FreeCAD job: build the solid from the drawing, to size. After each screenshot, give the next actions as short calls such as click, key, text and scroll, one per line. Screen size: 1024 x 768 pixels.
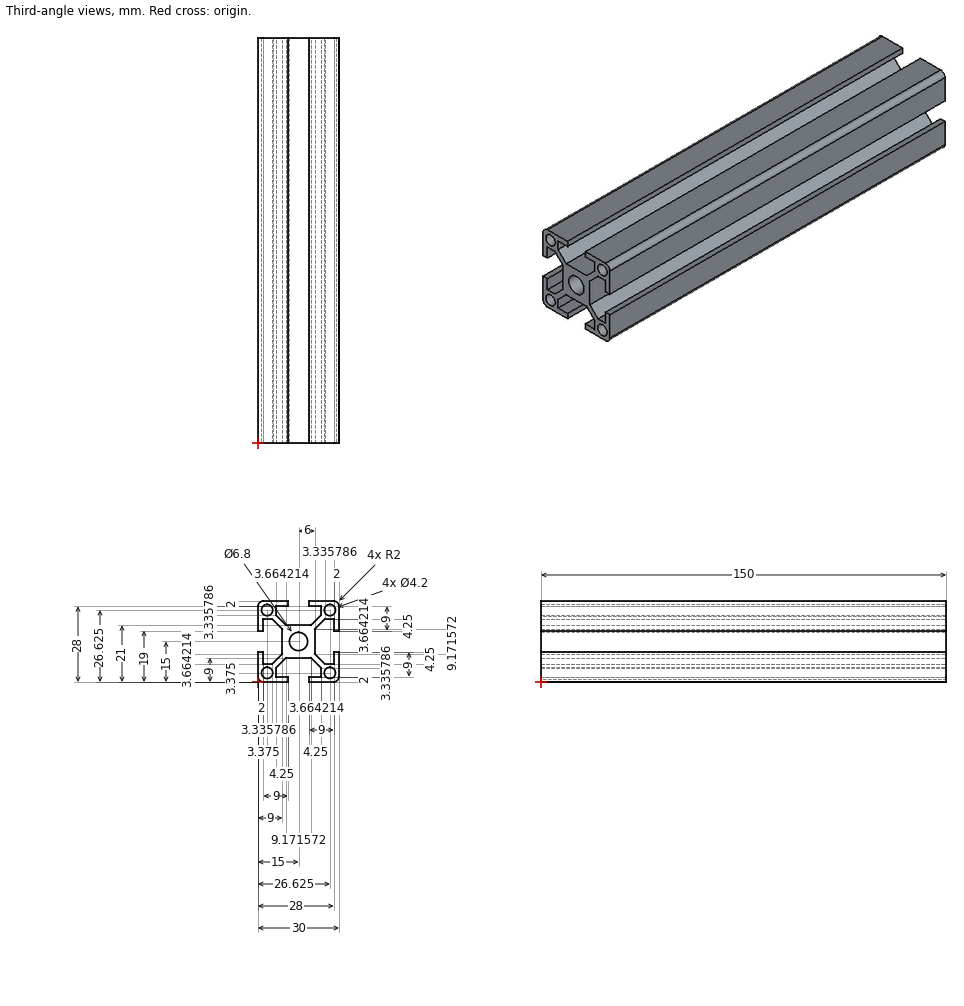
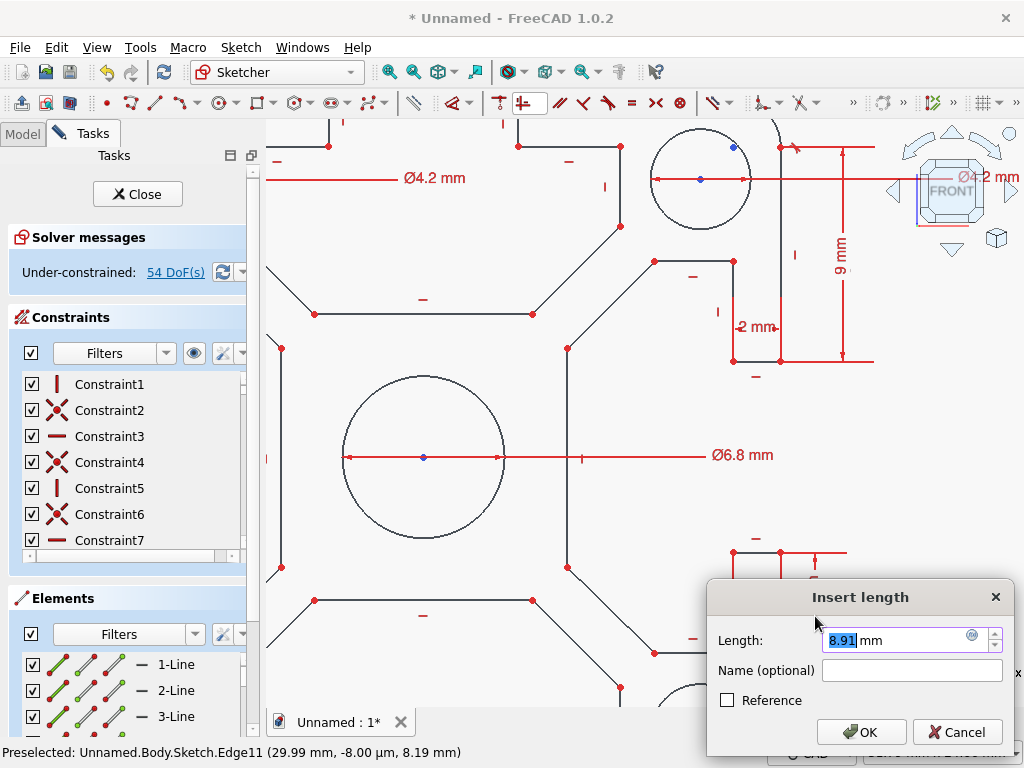
text(9)
key(Return)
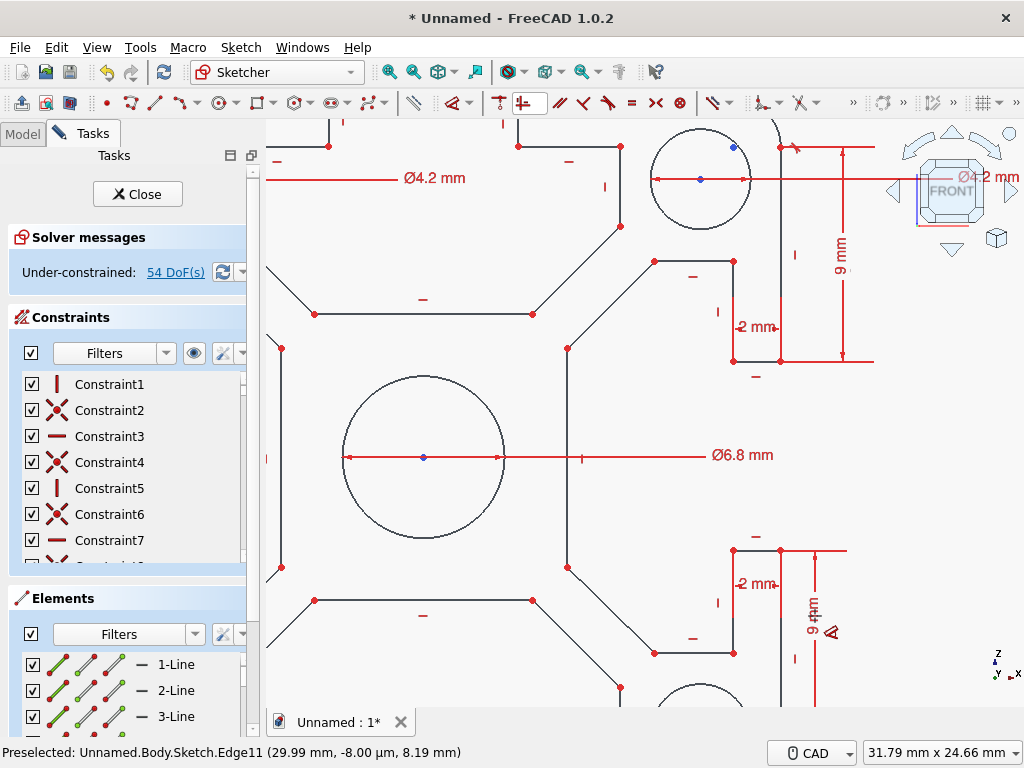
scroll(763, 361, down, 3)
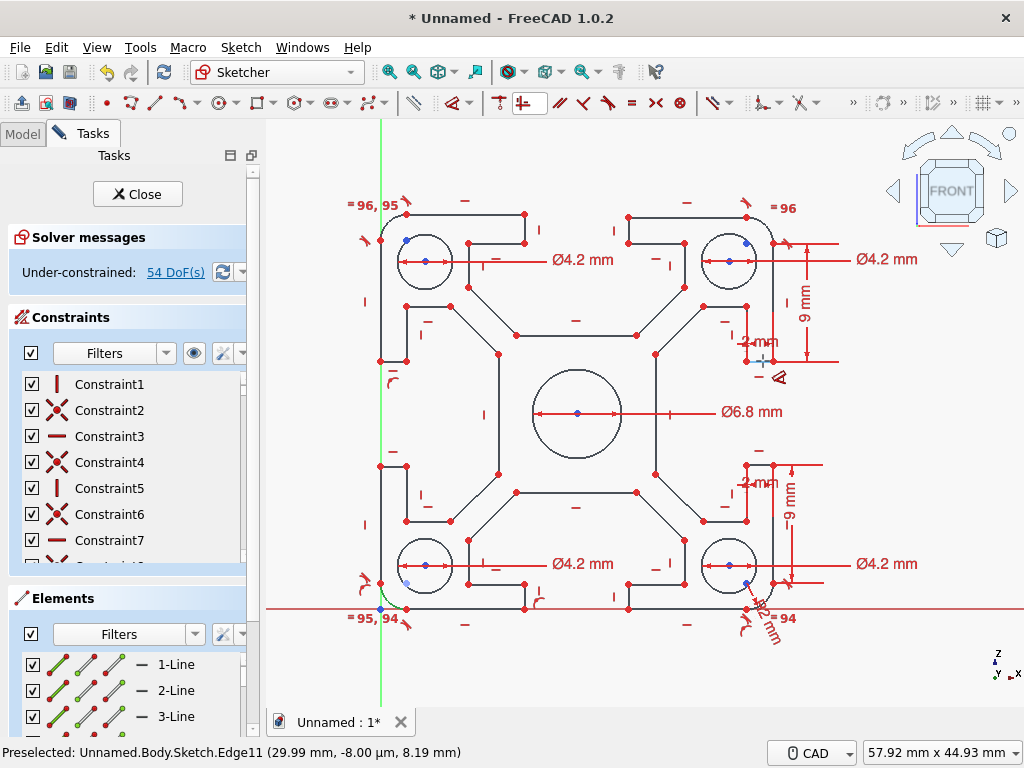
click(711, 609)
click(688, 643)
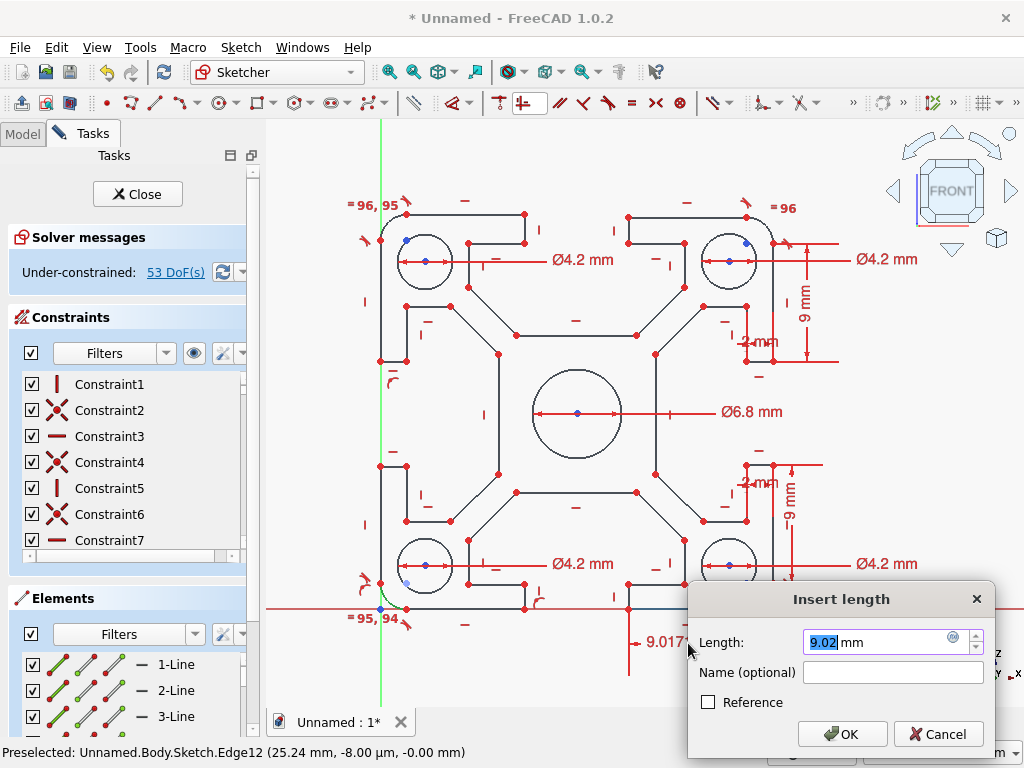
text(9)
key(Return)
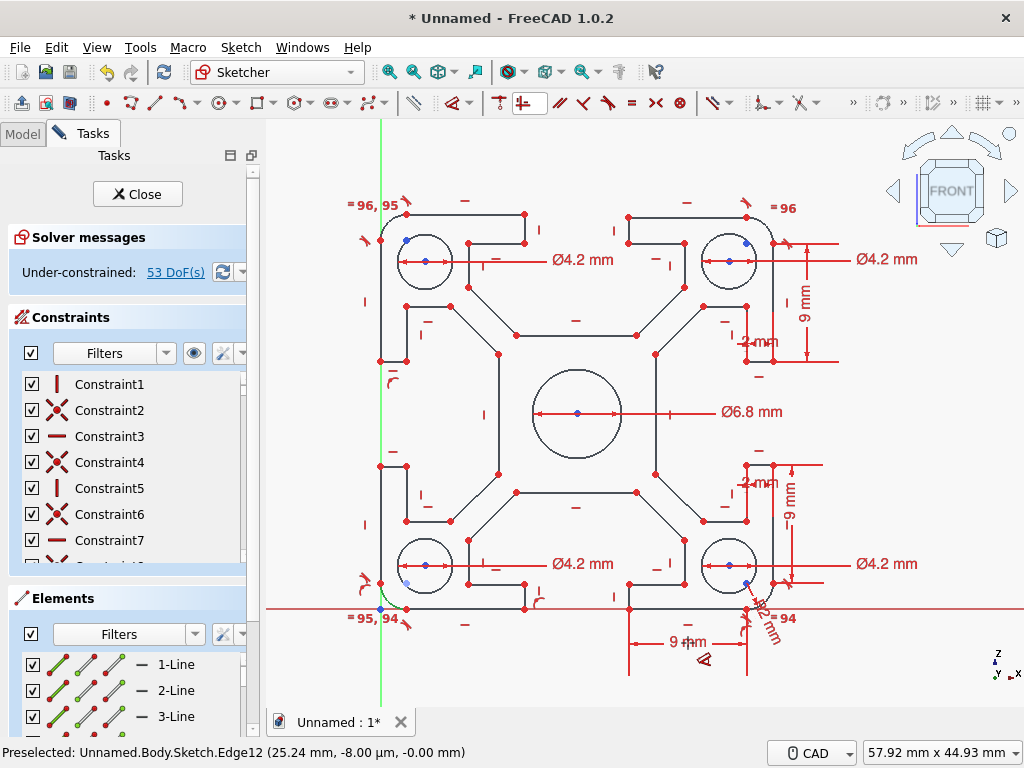
scroll(629, 599, up, 3)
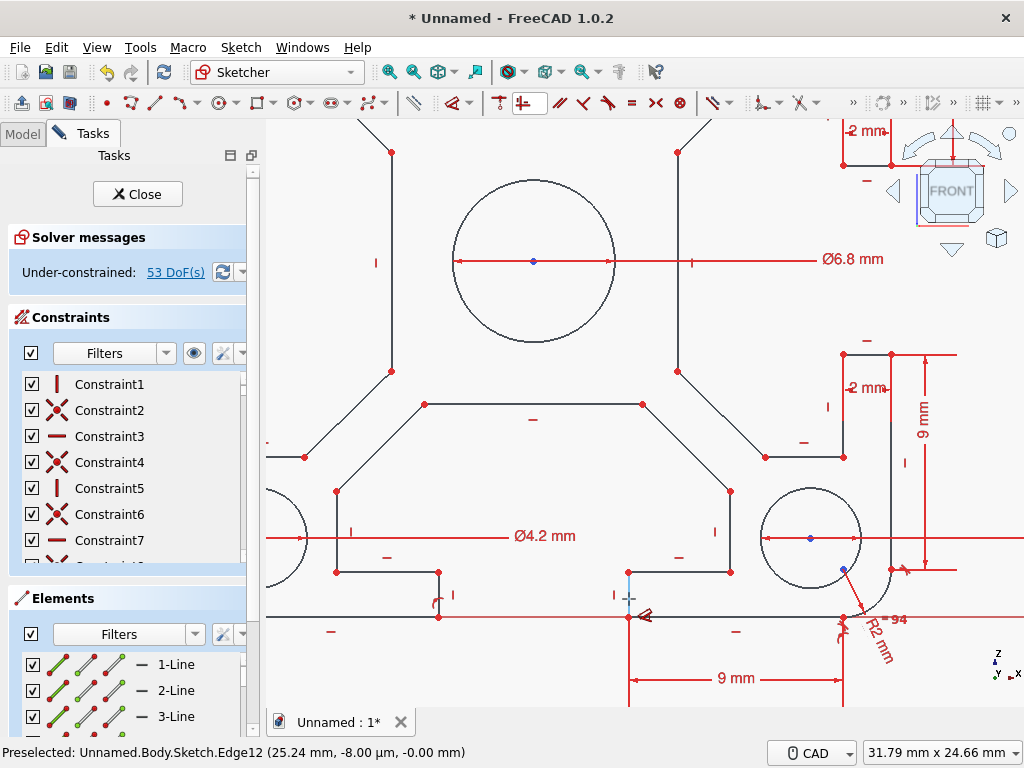
click(629, 599)
click(663, 595)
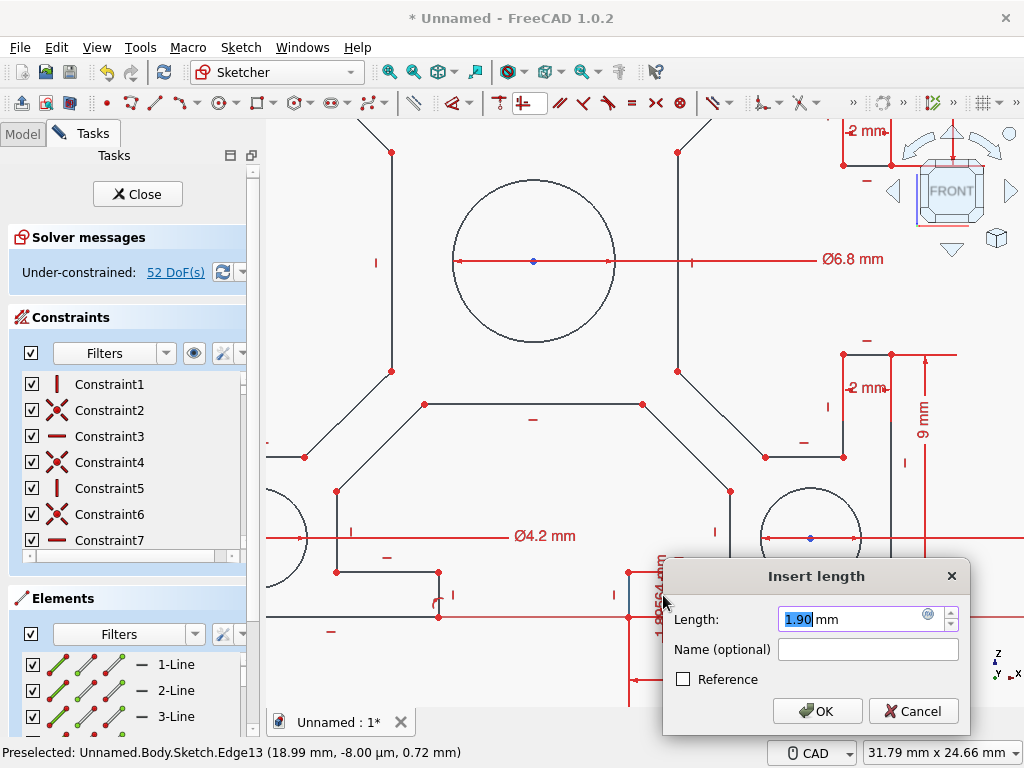
text(2)
key(Return)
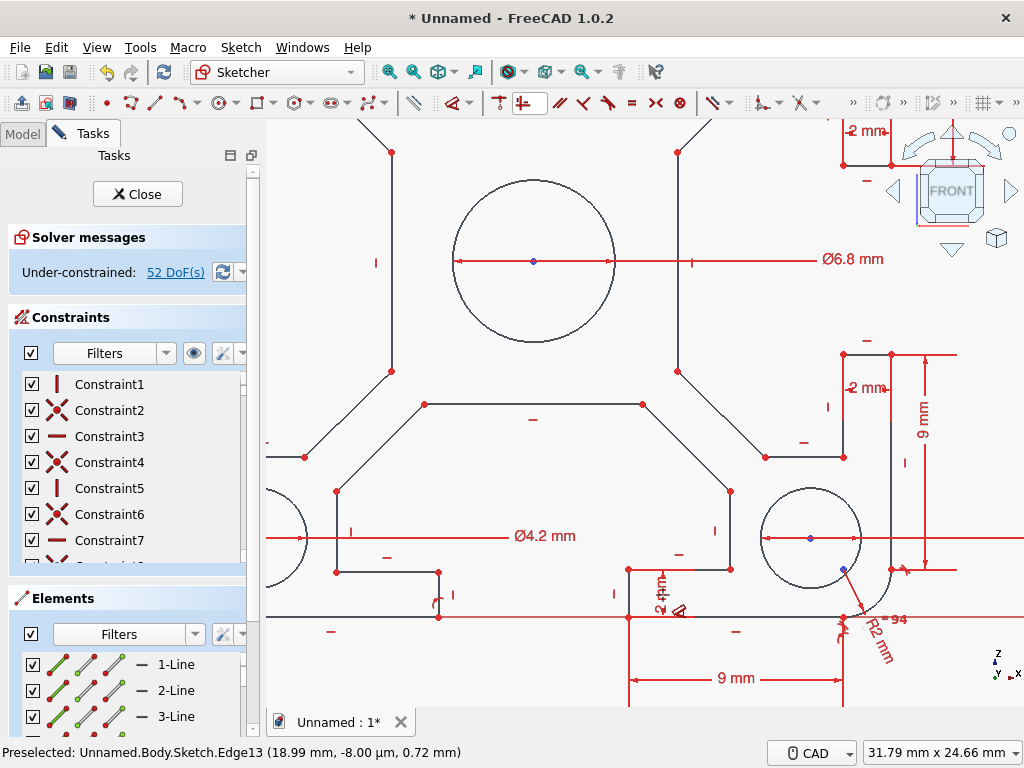
click(439, 586)
click(405, 595)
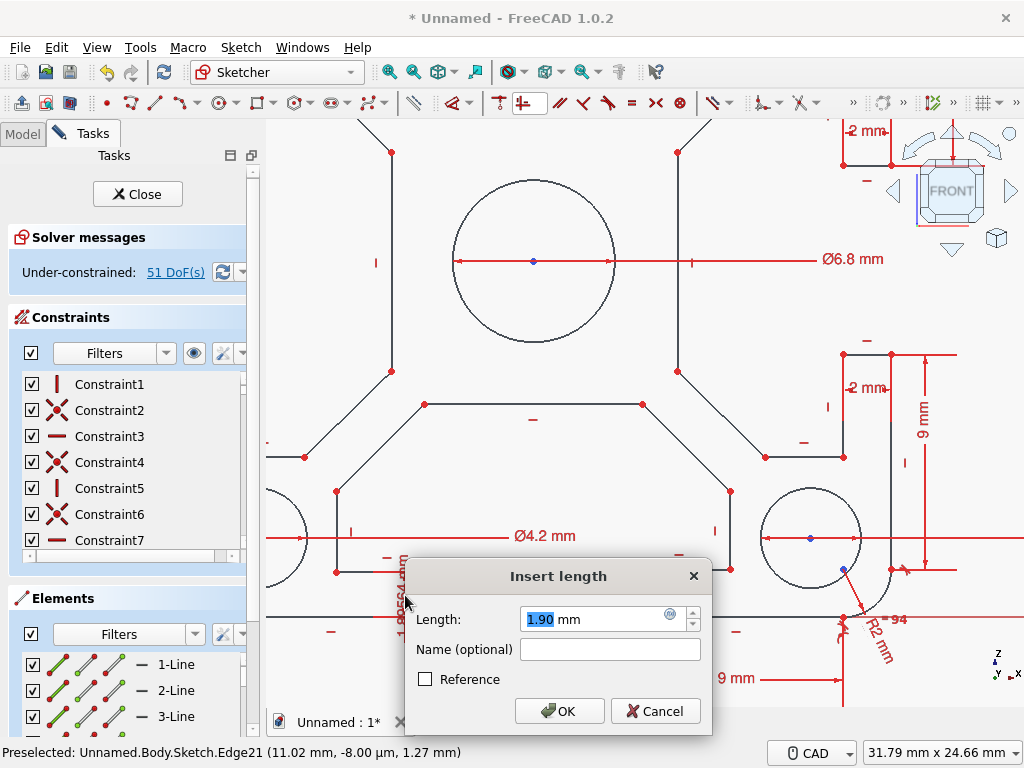
text(2)
key(Return)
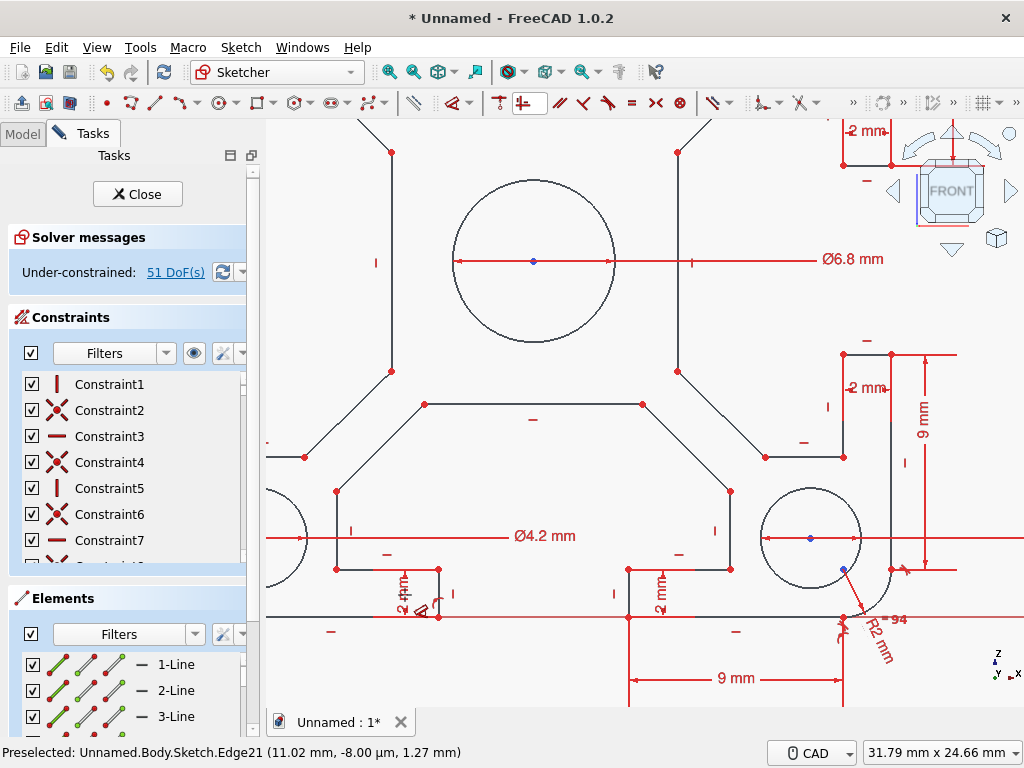
click(374, 617)
click(366, 651)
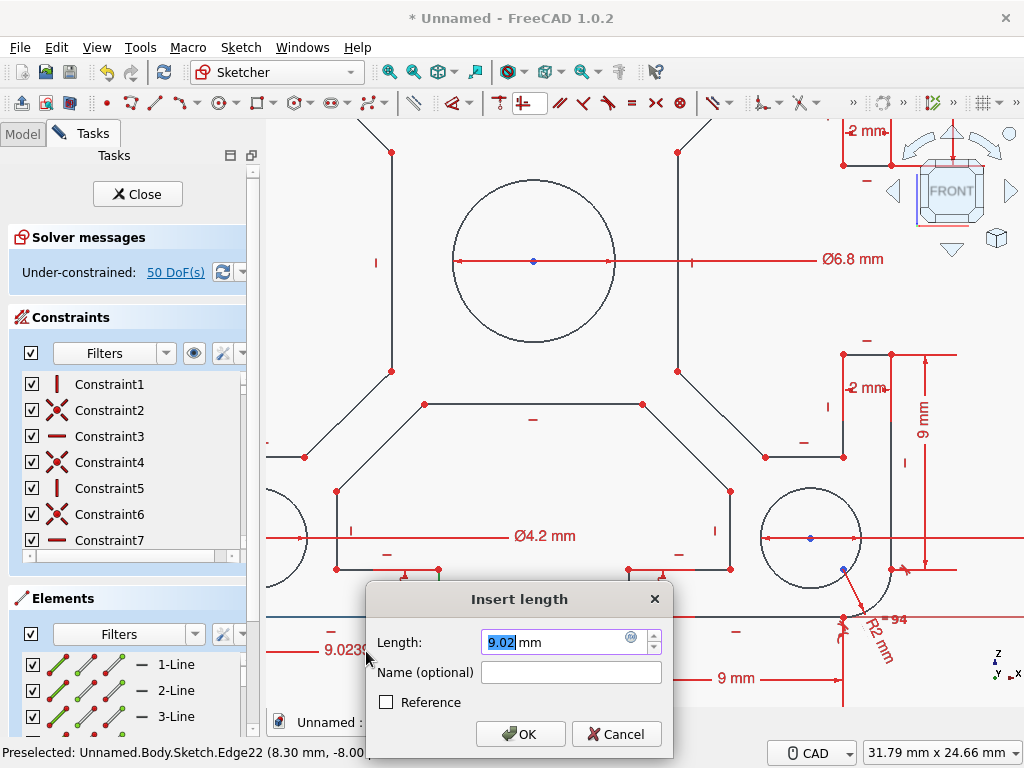
text(9)
key(Return)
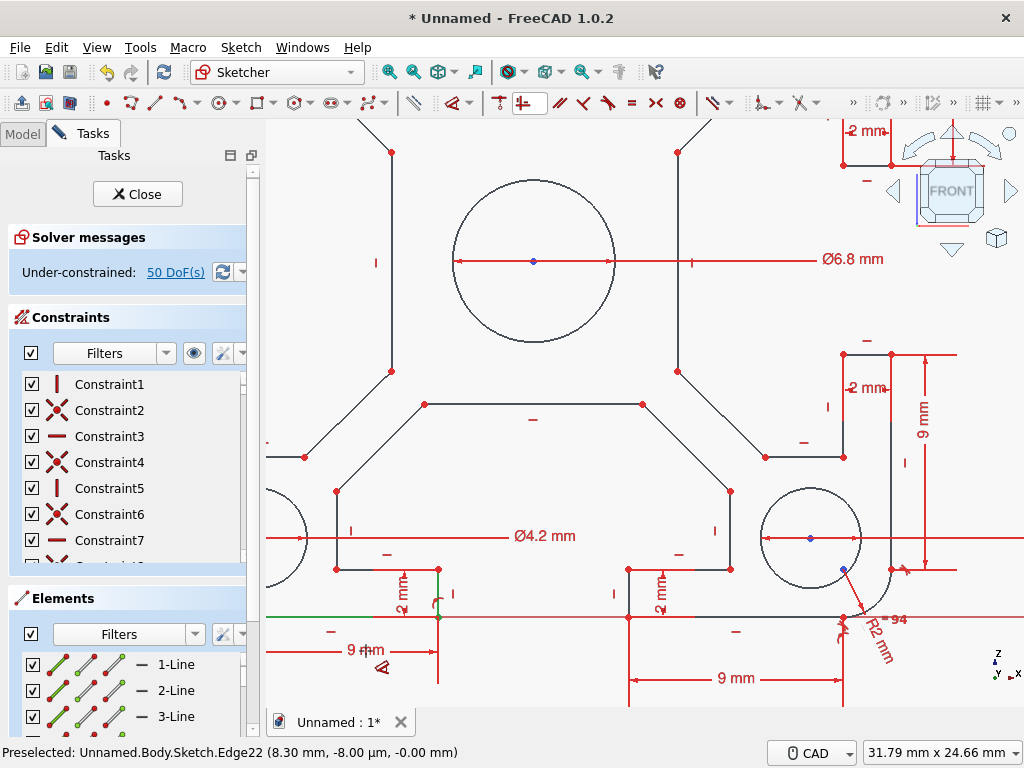
scroll(628, 600, down, 3)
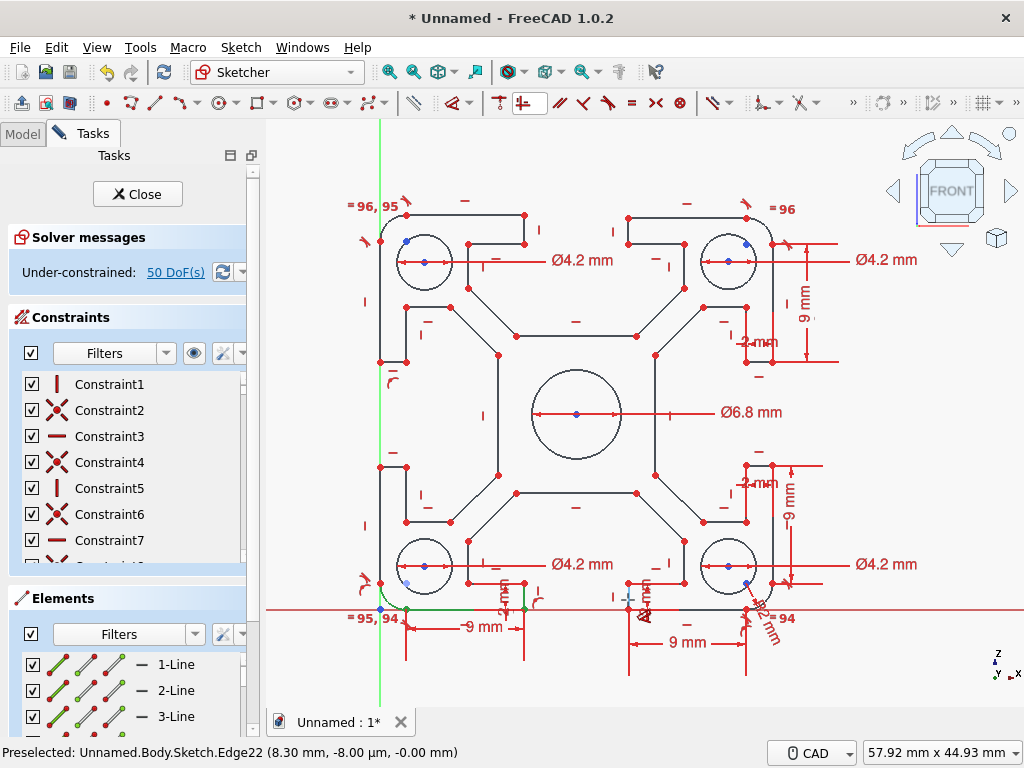
click(380, 549)
click(346, 525)